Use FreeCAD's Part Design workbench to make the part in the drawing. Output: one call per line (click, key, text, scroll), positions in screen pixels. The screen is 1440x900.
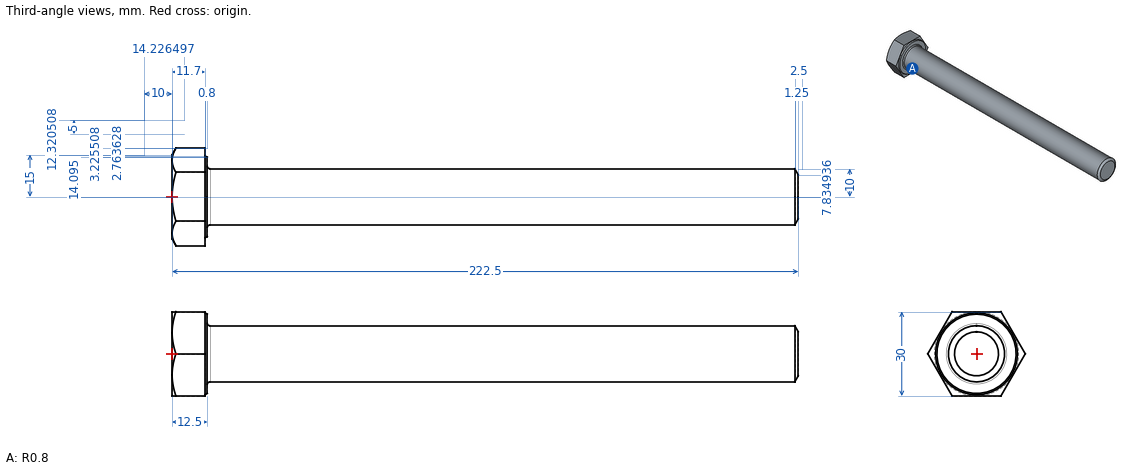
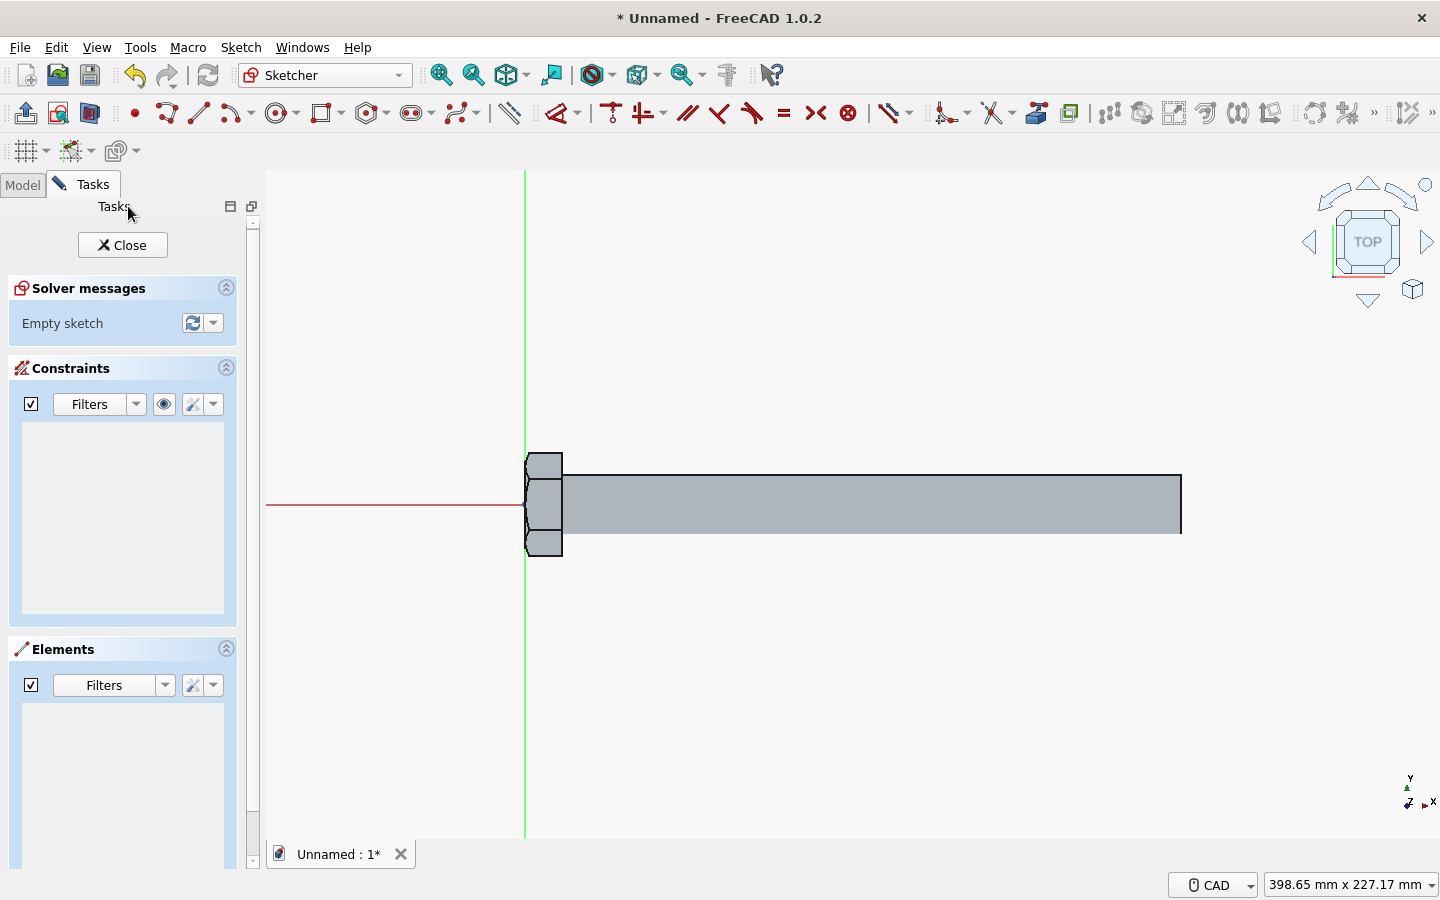
click(90, 114)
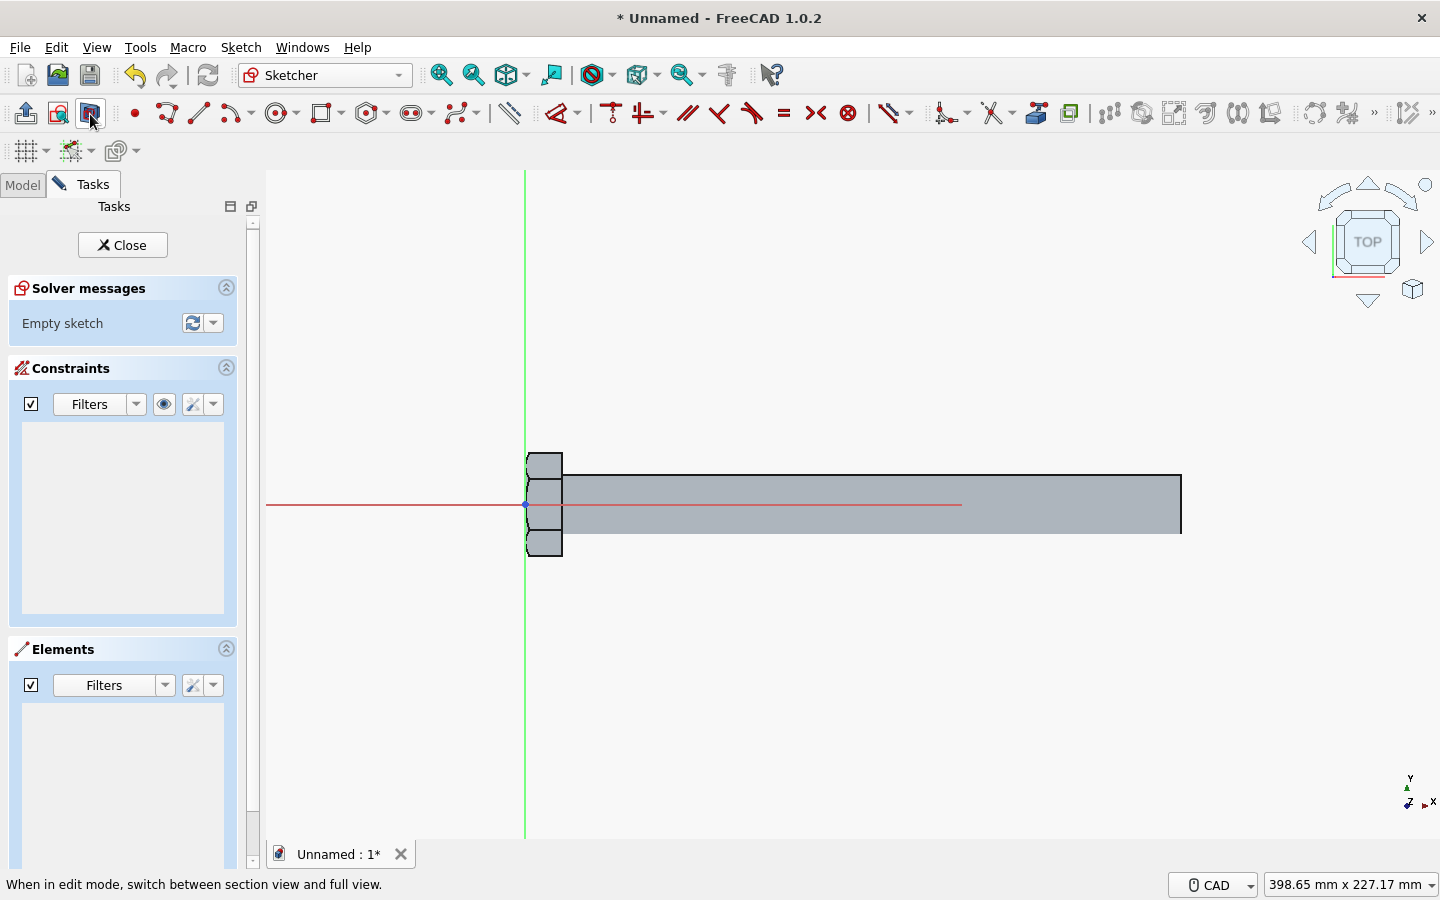
scroll(549, 456, up, 15)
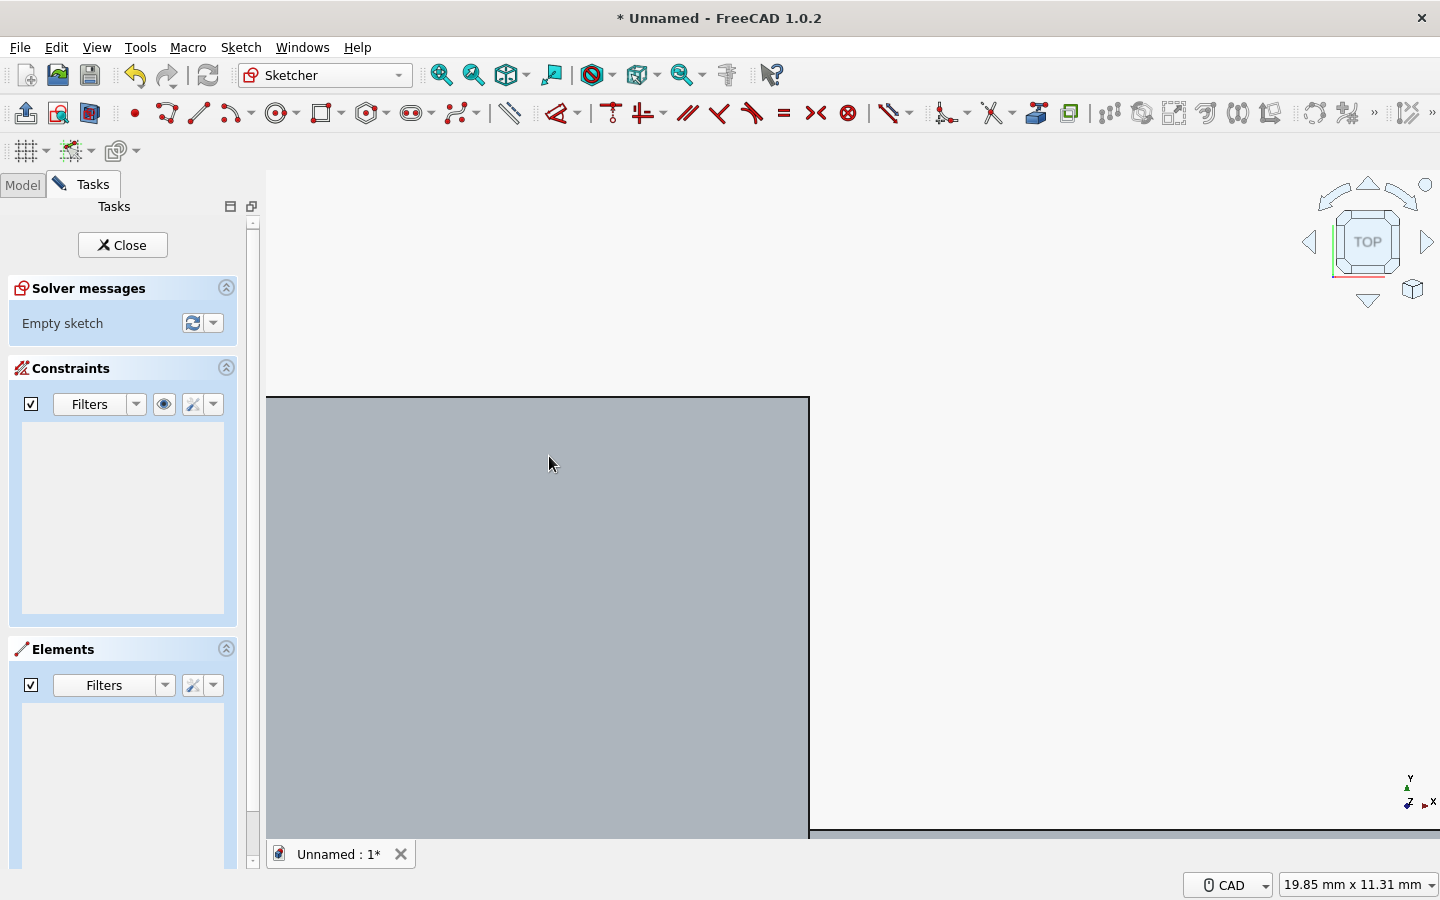
scroll(787, 483, up, 4)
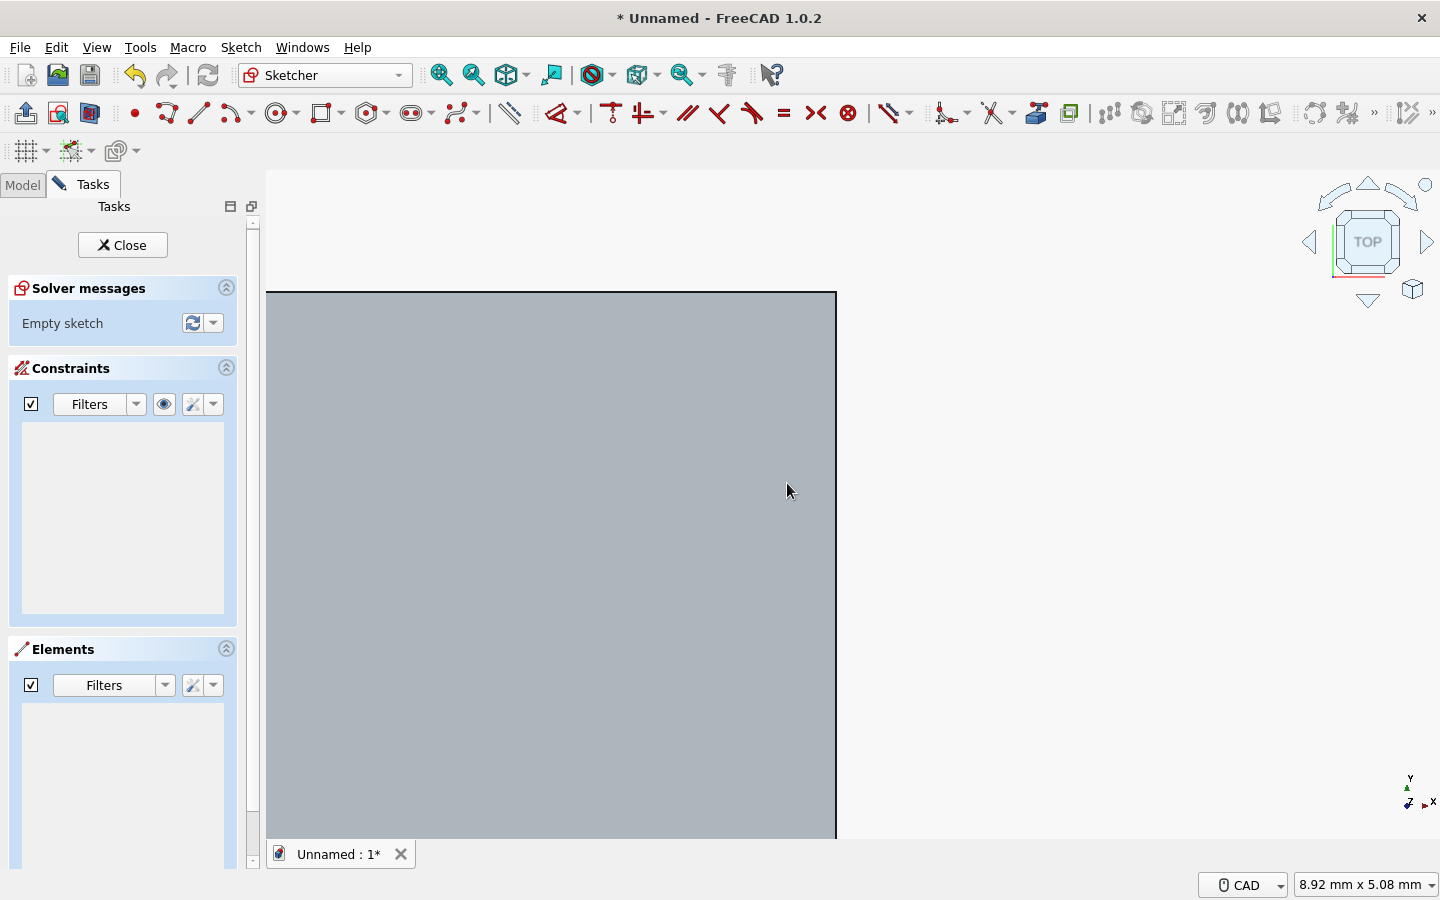
click(168, 114)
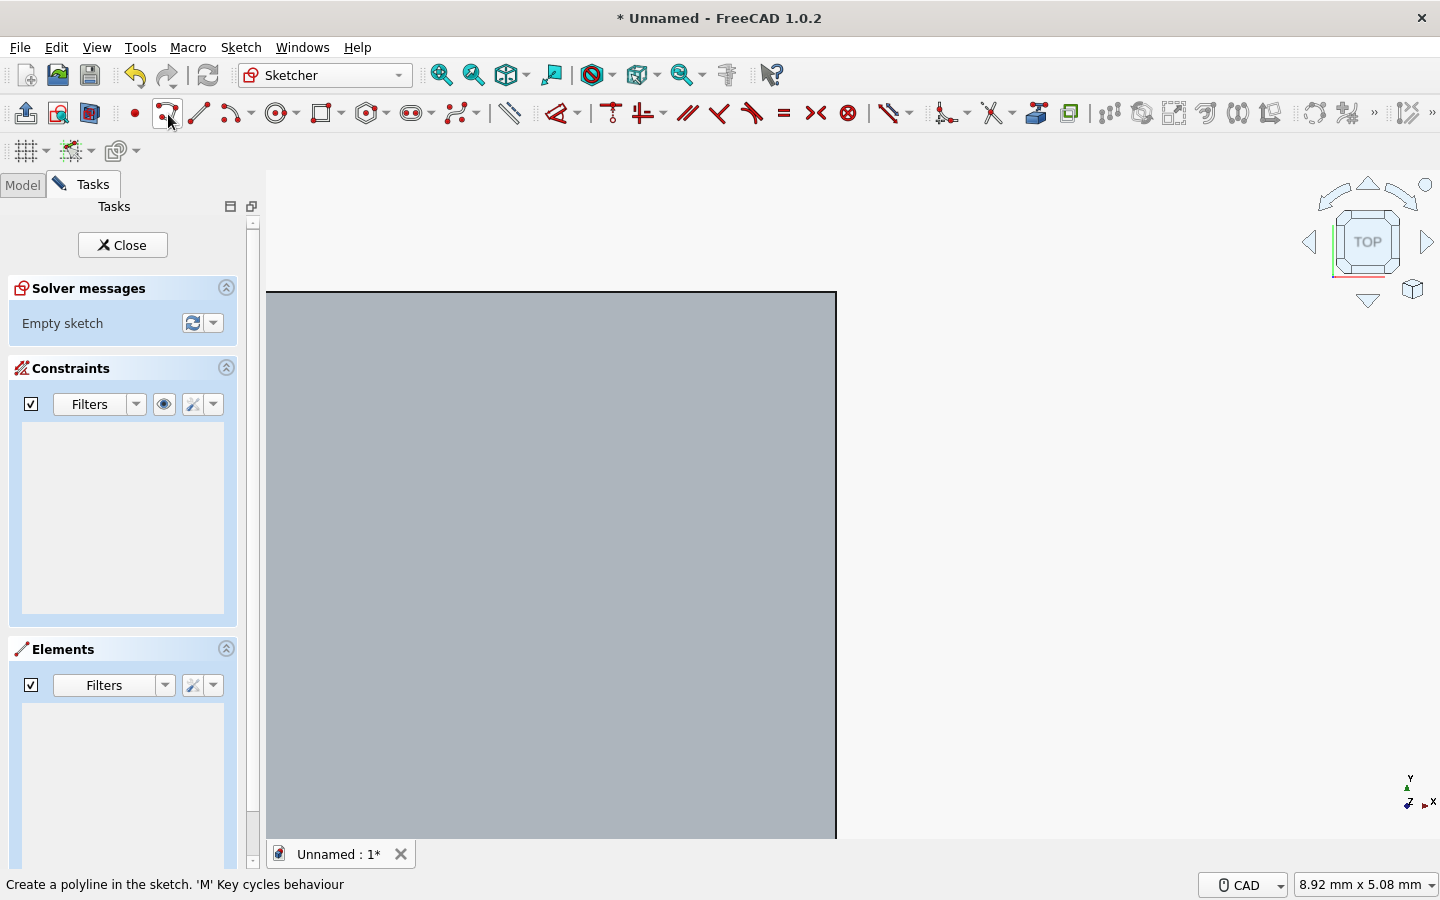
click(731, 656)
click(836, 717)
click(836, 292)
click(731, 292)
click(731, 657)
key(Escape)
key(Escape)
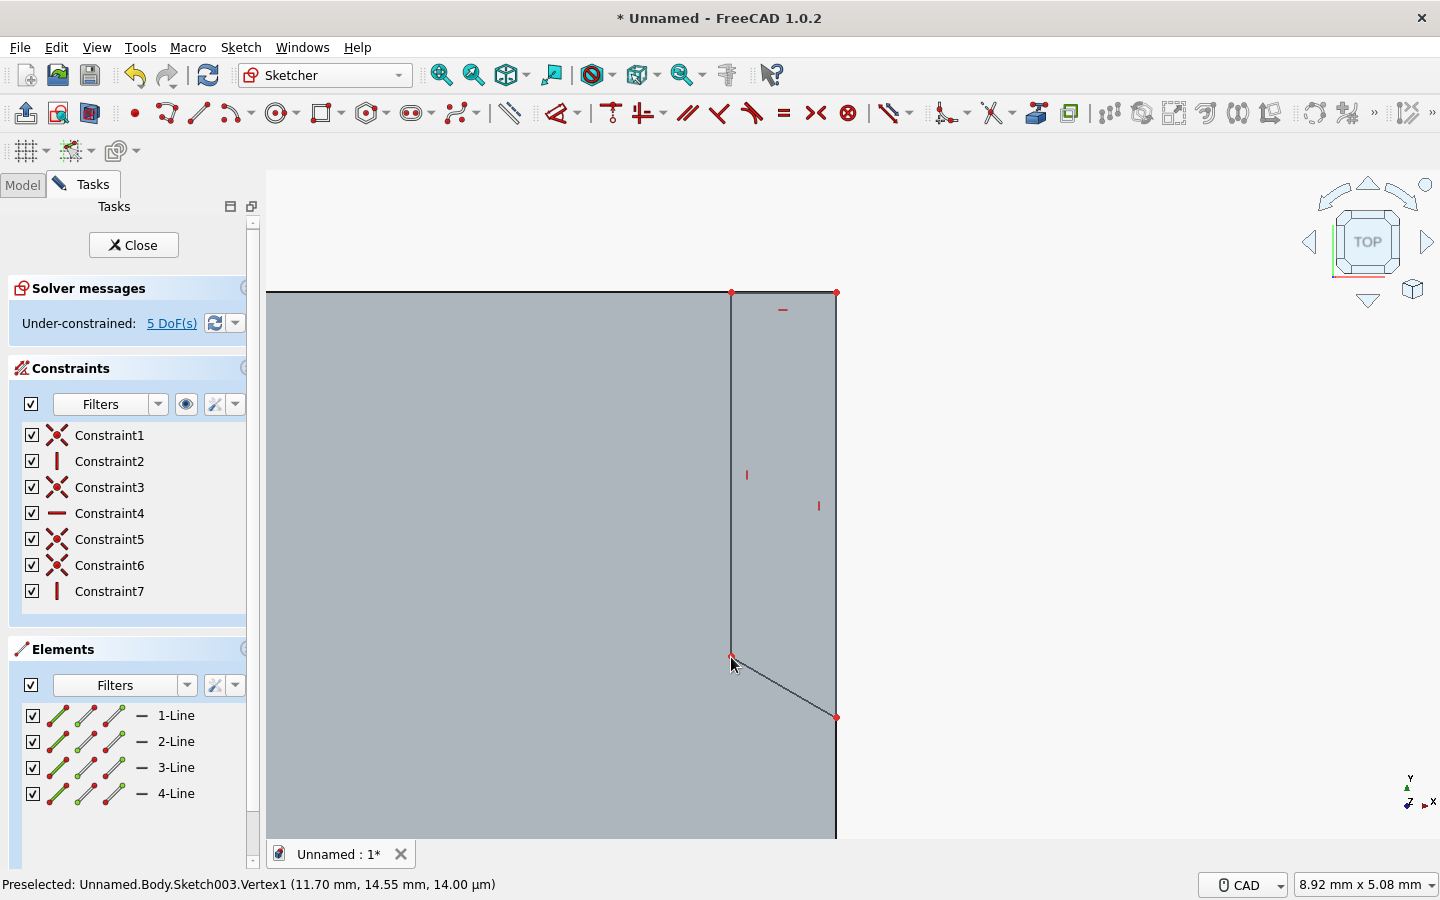
click(556, 114)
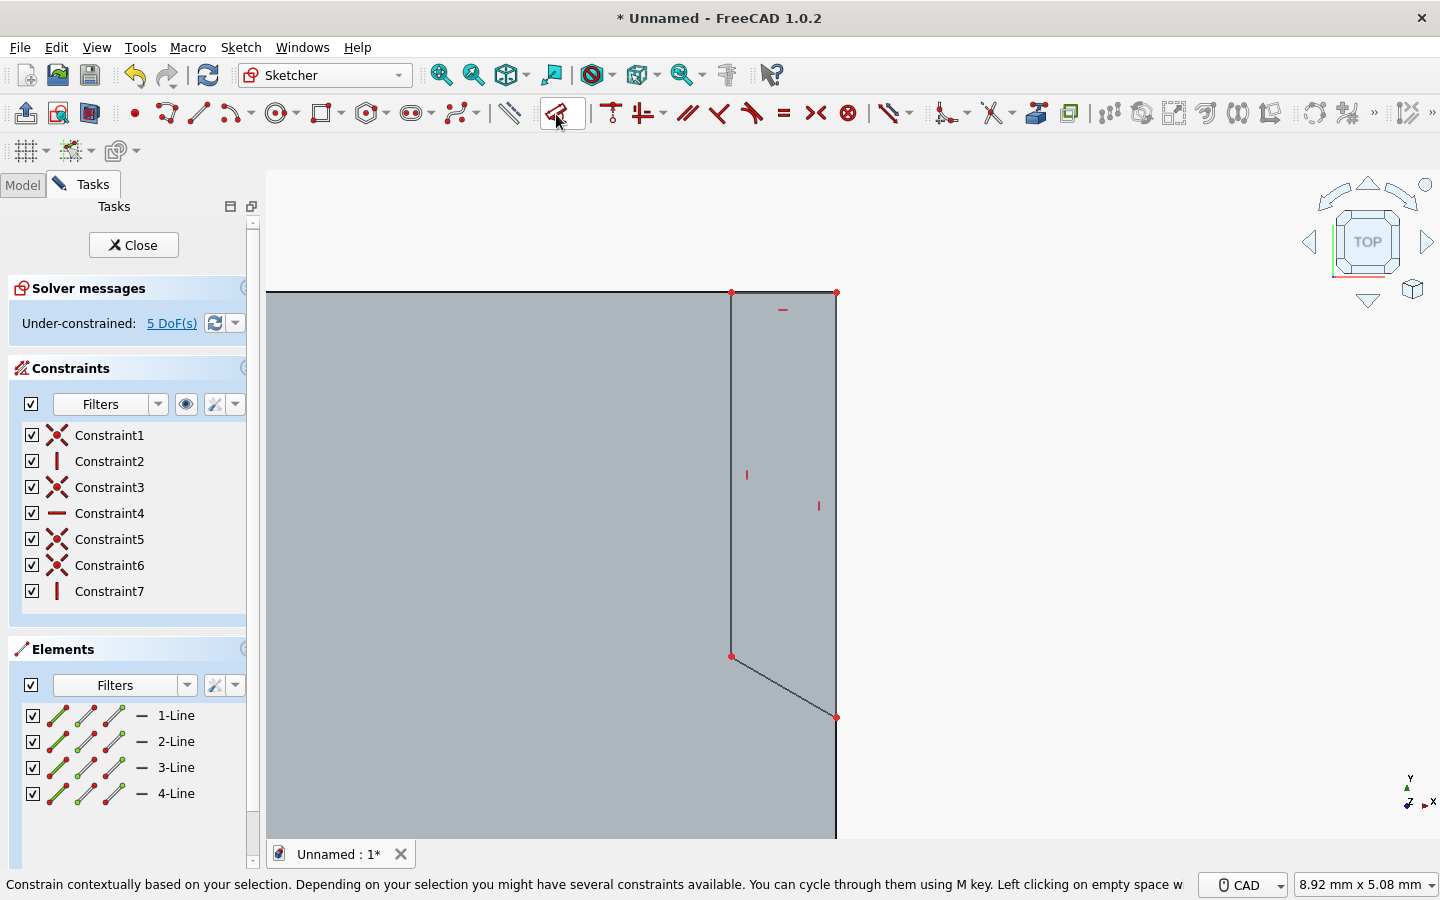
click(805, 293)
click(784, 259)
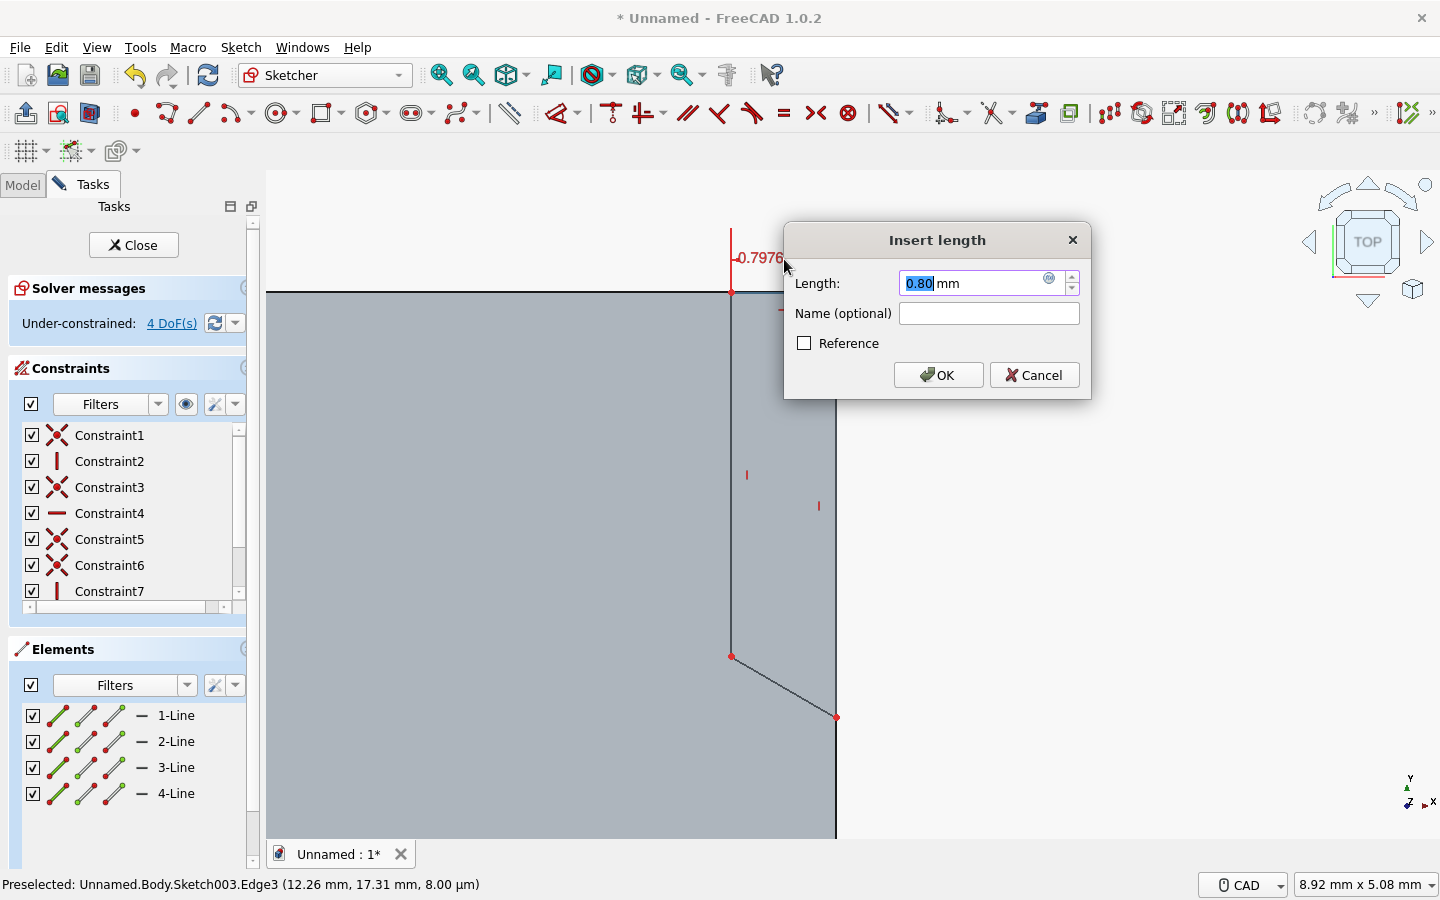
text(0.8)
key(Return)